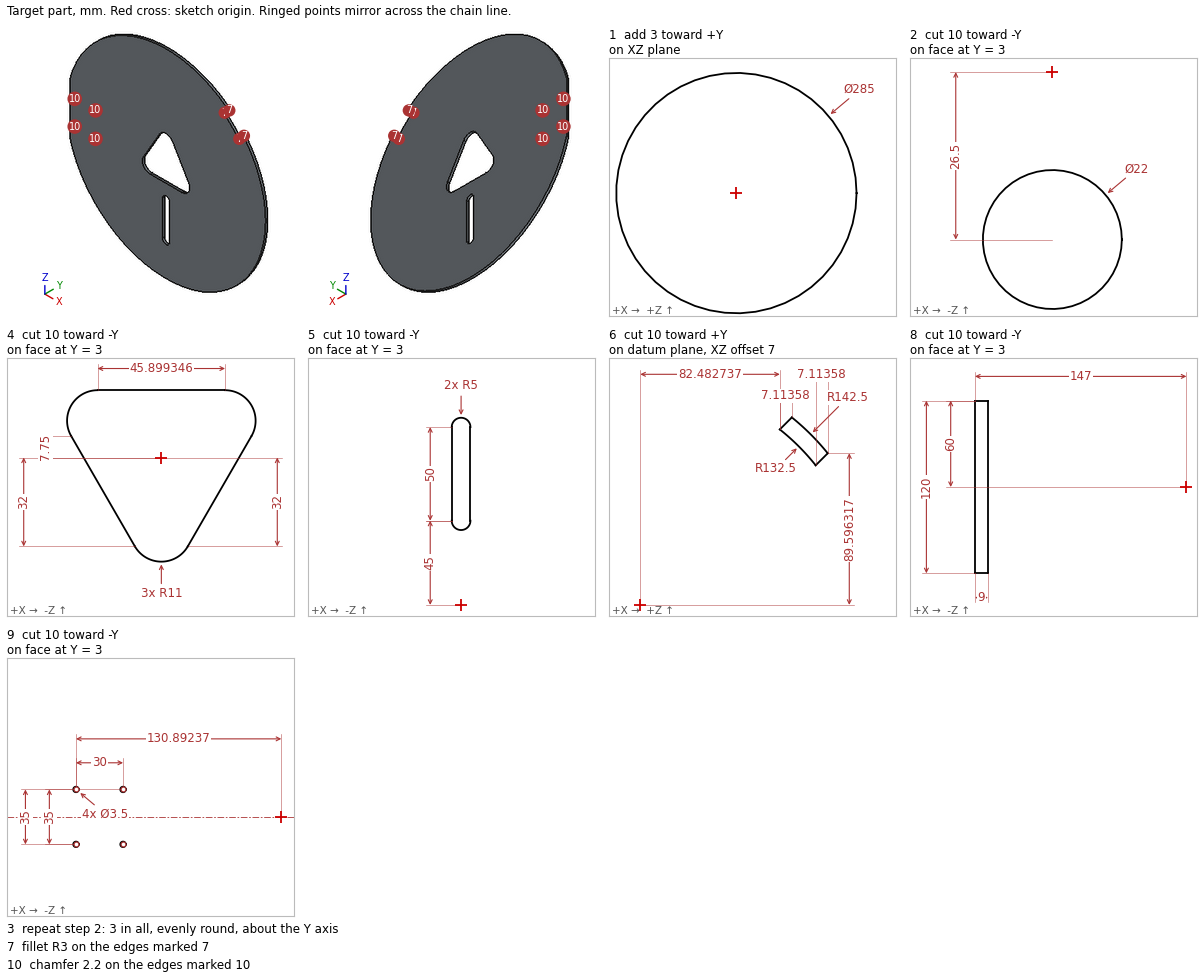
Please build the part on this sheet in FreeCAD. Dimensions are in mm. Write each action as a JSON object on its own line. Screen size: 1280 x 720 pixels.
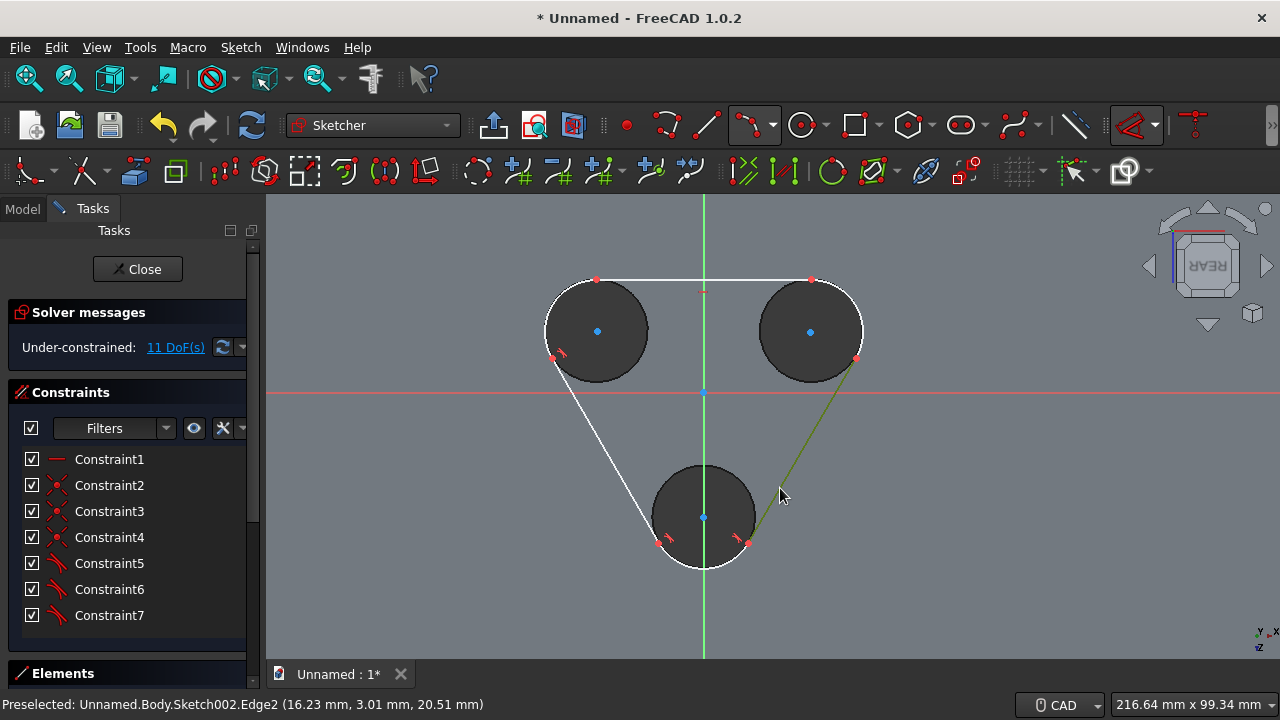
{"action": "left_click", "coordinate": [863, 327]}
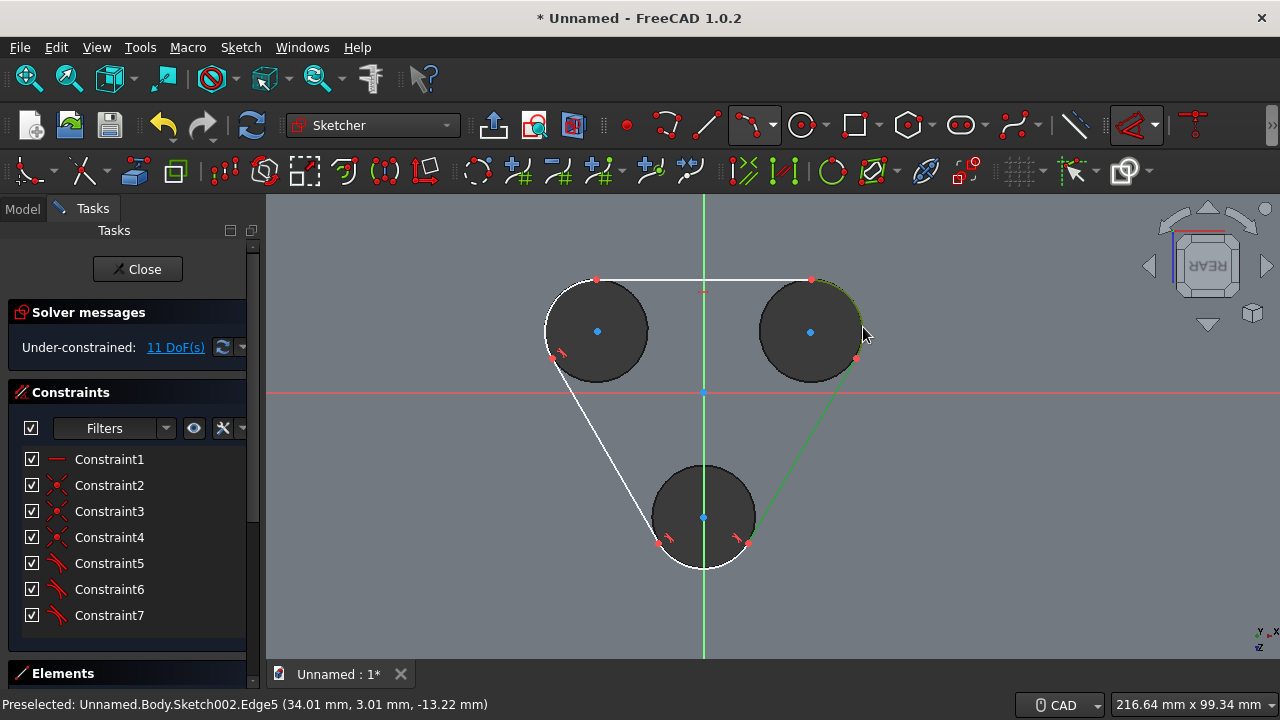
{"action": "key", "text": "t"}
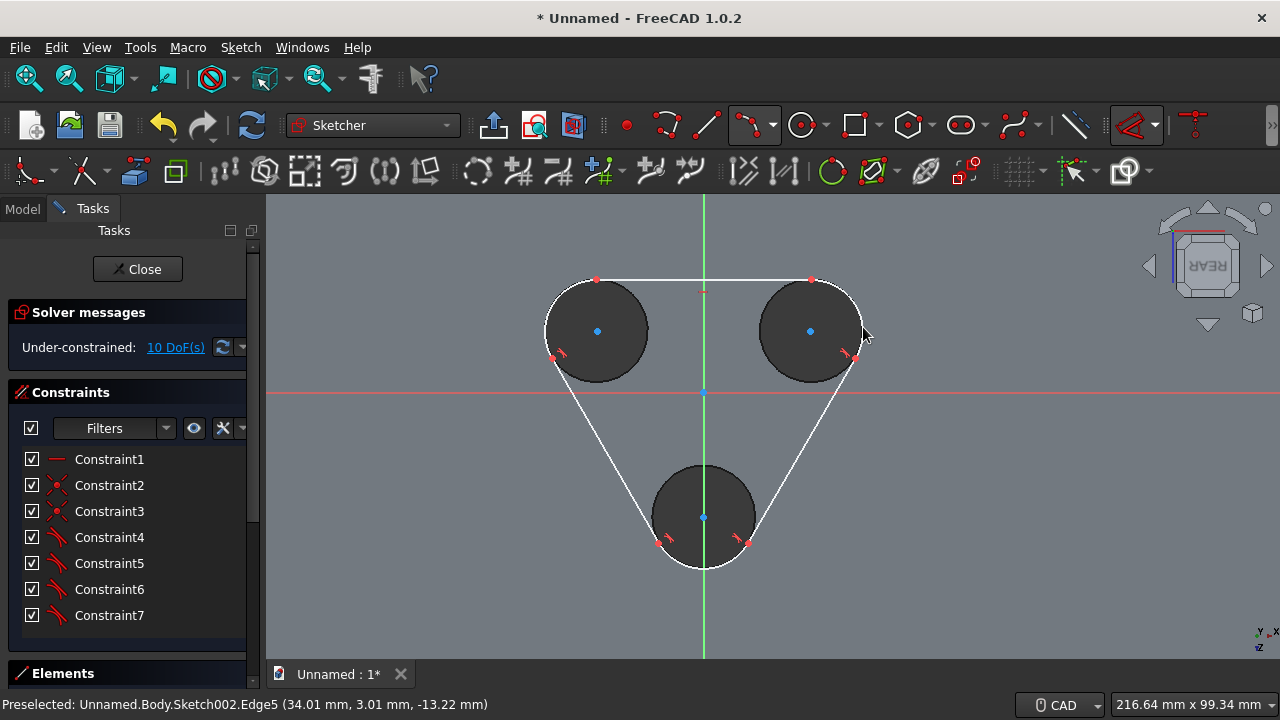
{"action": "left_click", "coordinate": [746, 280]}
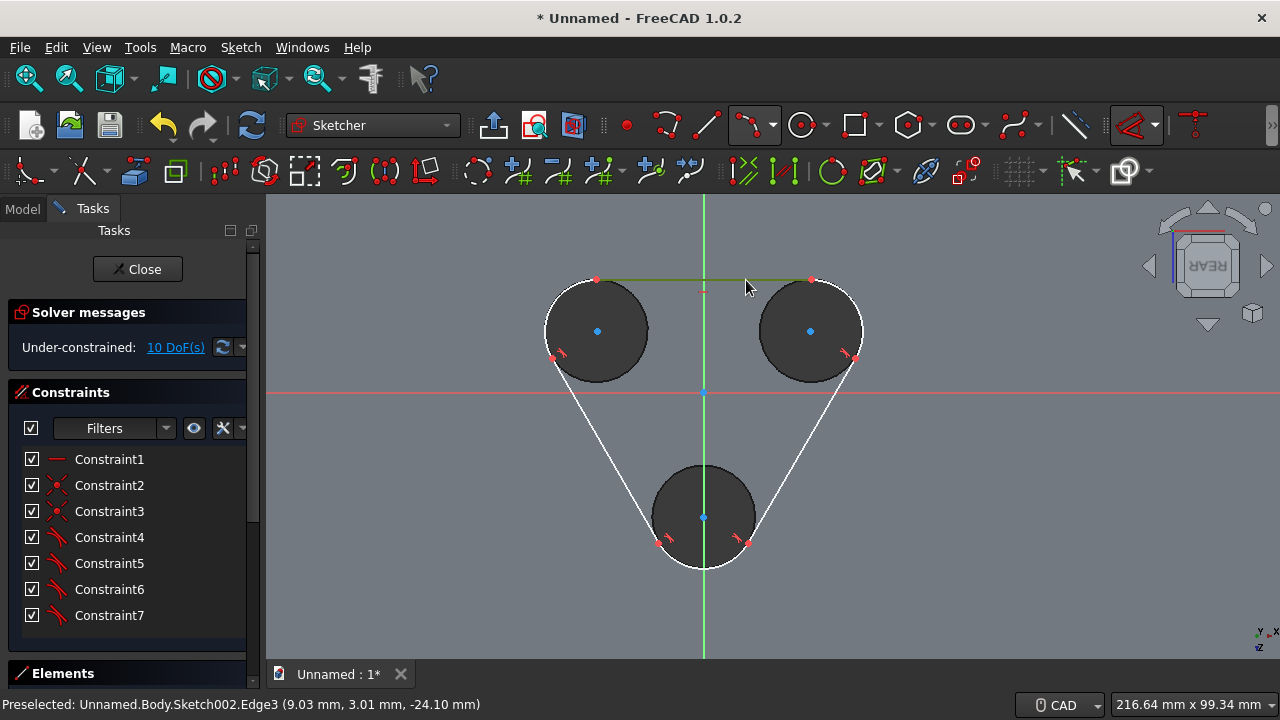
{"action": "left_click", "coordinate": [863, 327]}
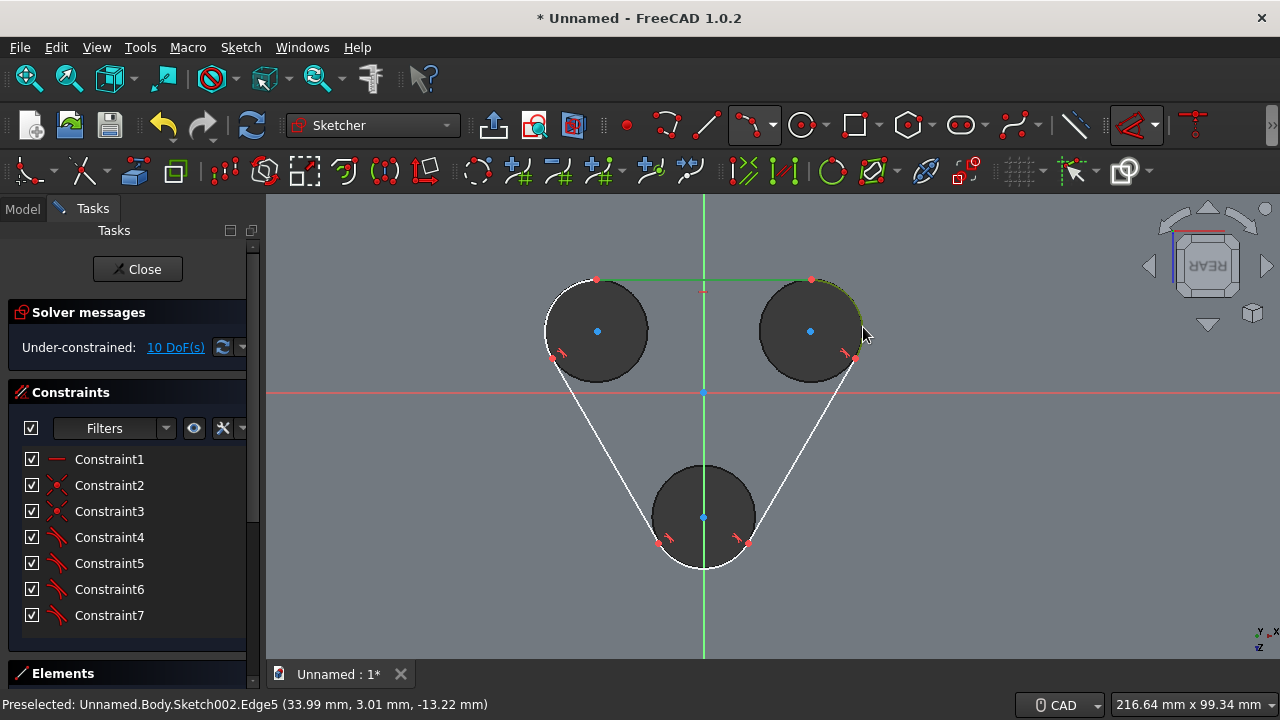
{"action": "key", "text": "t"}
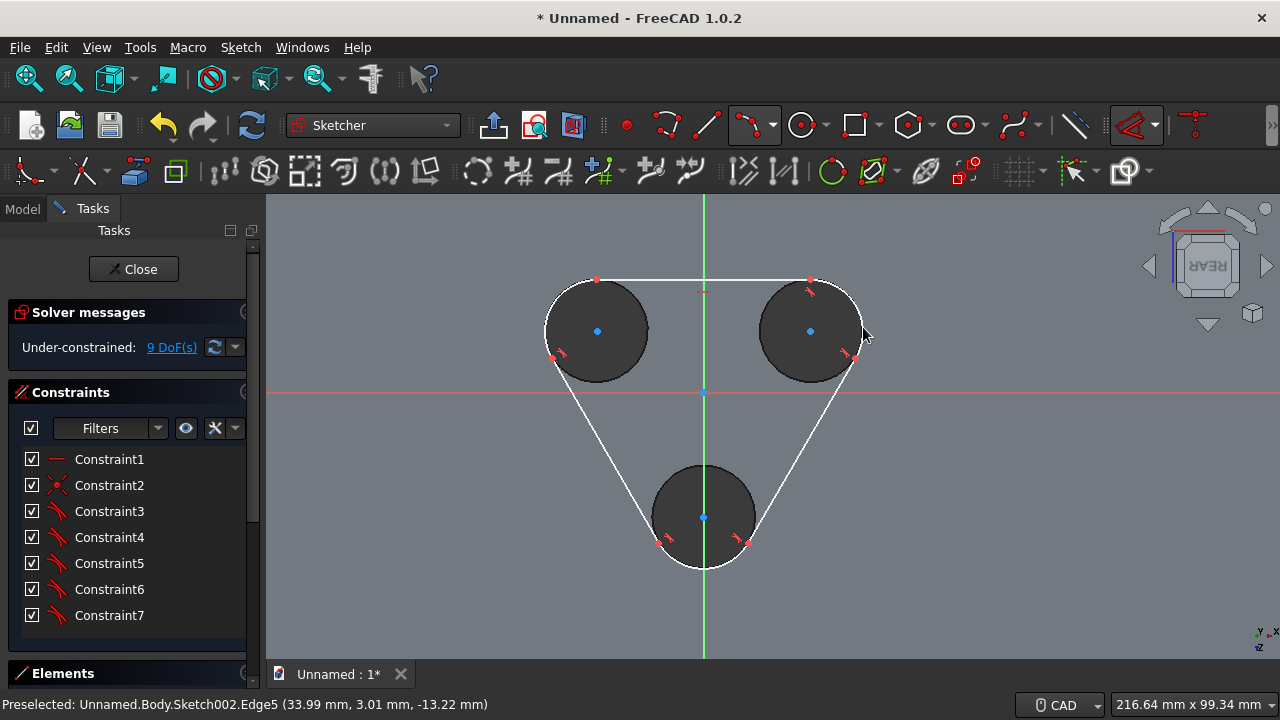
{"action": "left_click", "coordinate": [746, 280]}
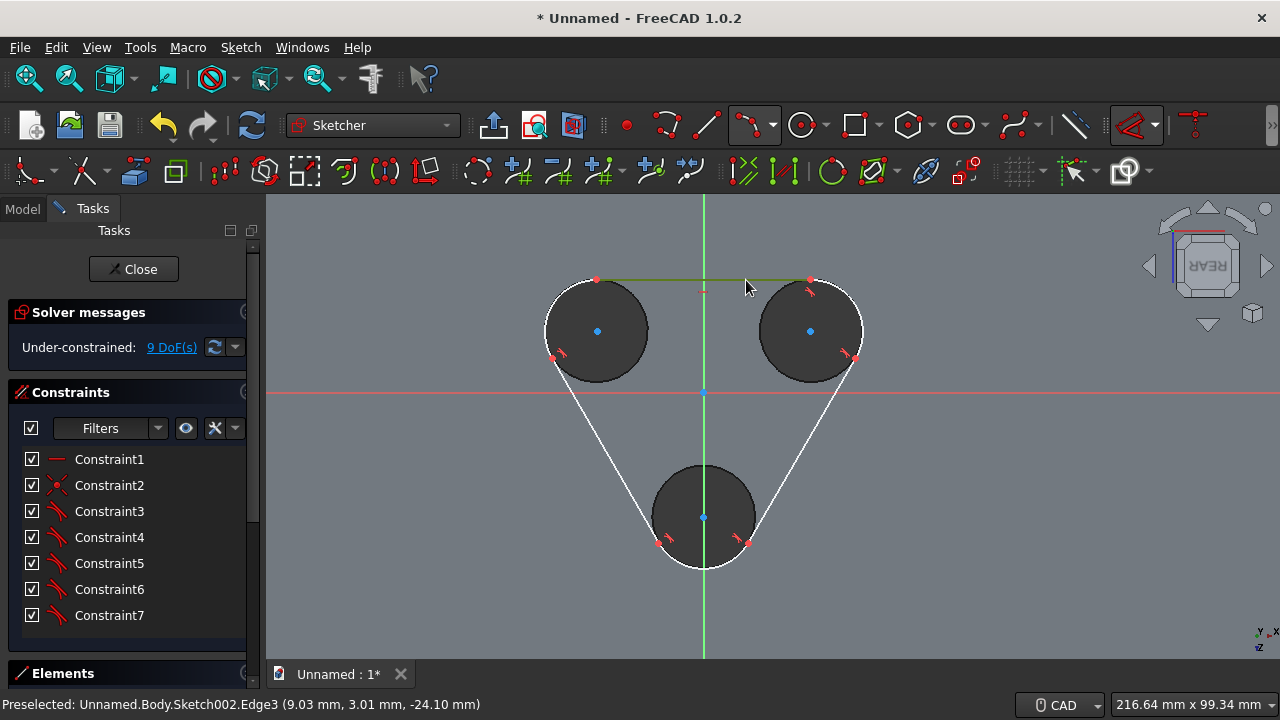
{"action": "left_click", "coordinate": [566, 290]}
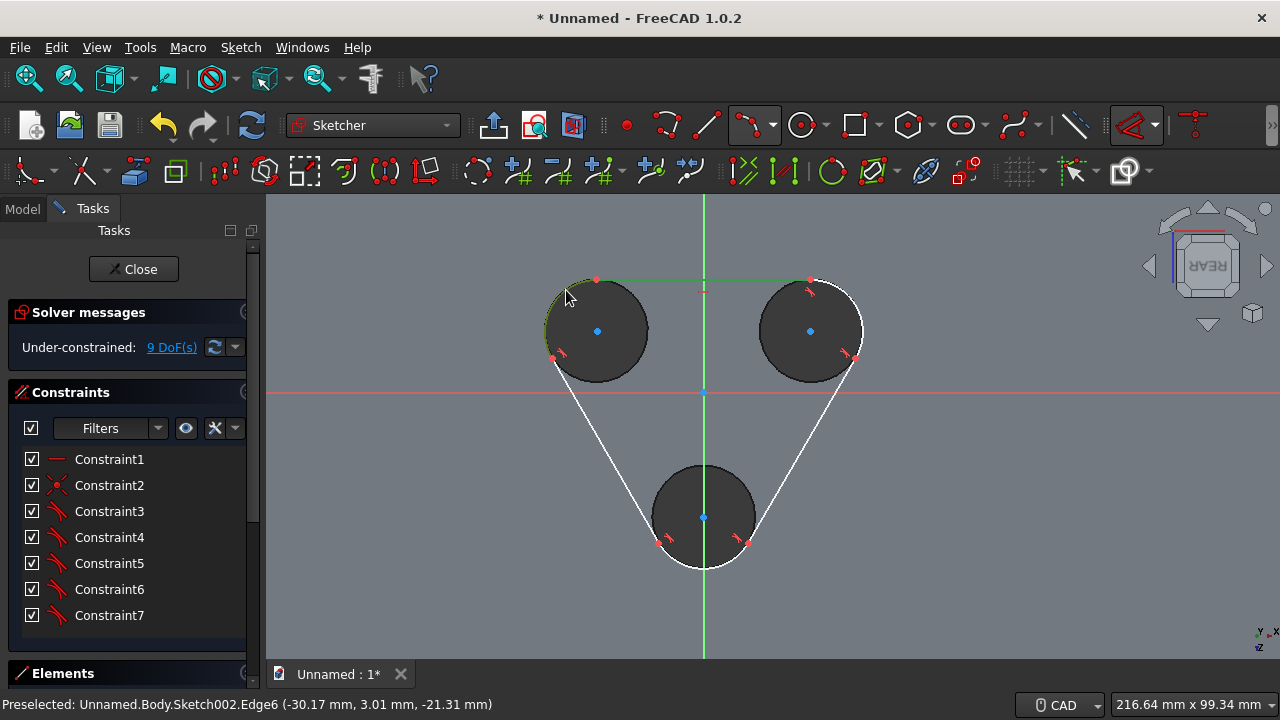
{"action": "key", "text": "t"}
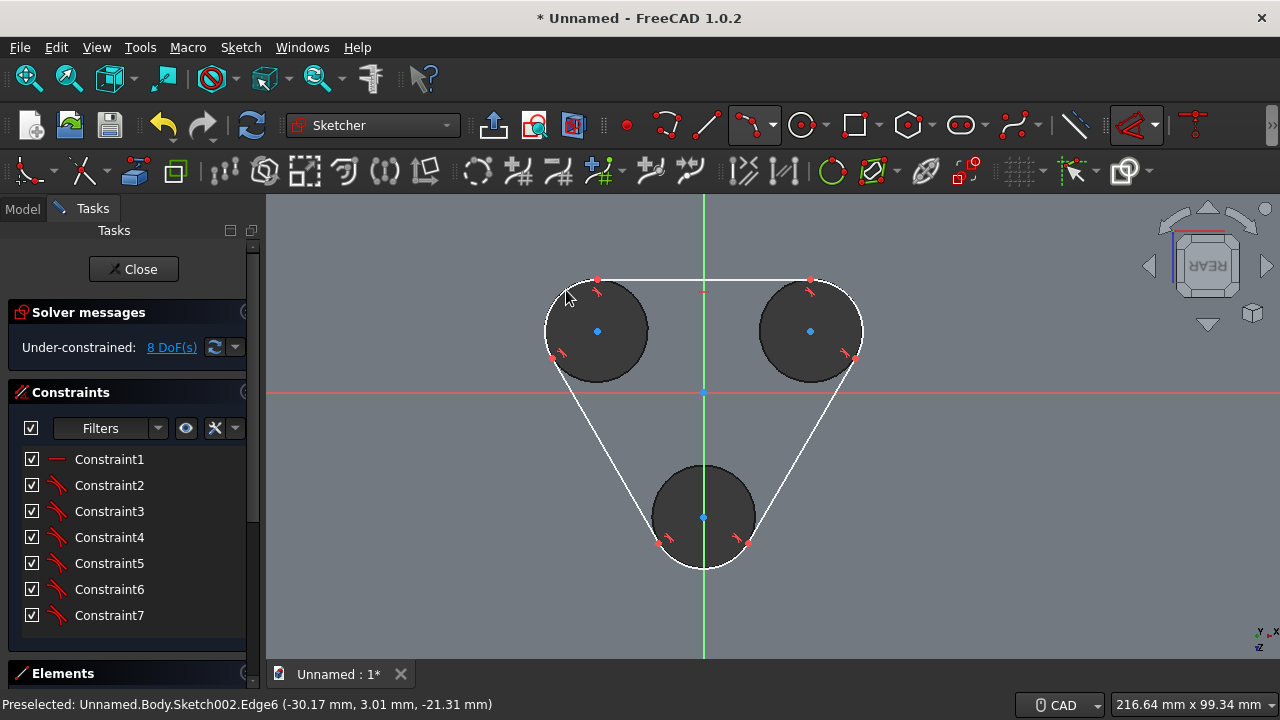
{"action": "left_click", "coordinate": [683, 564]}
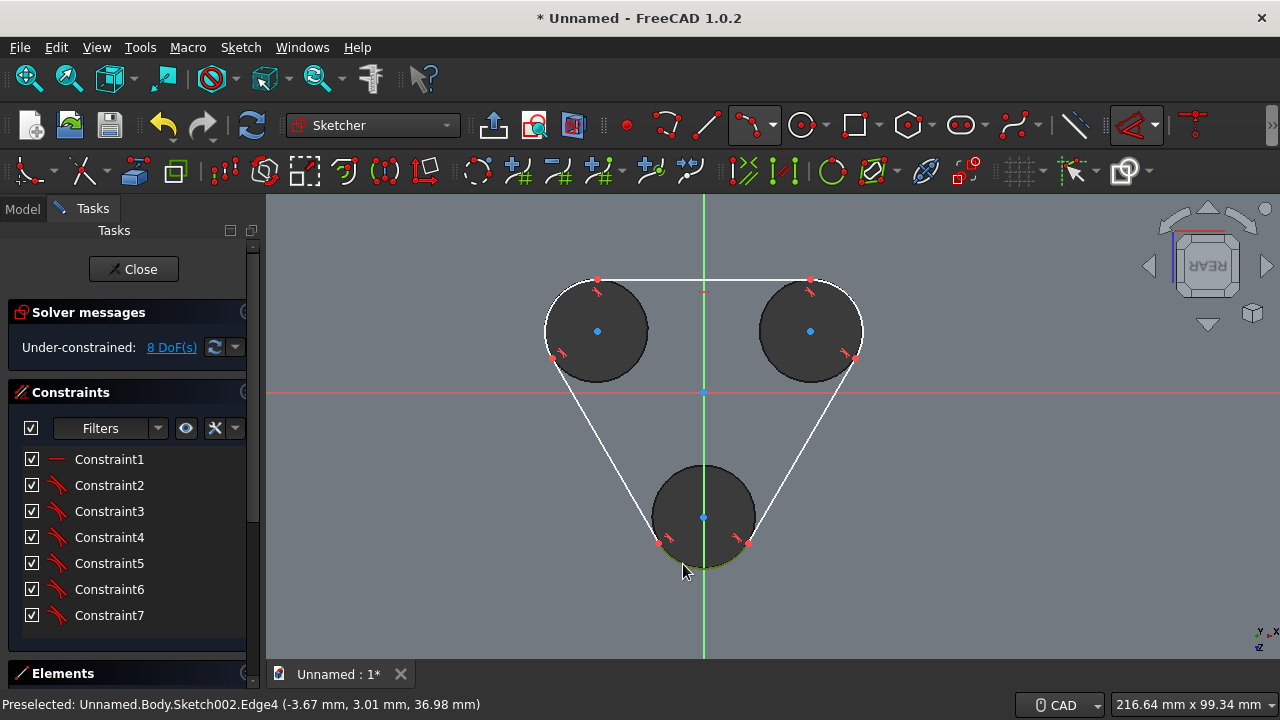
{"action": "left_click", "coordinate": [863, 327]}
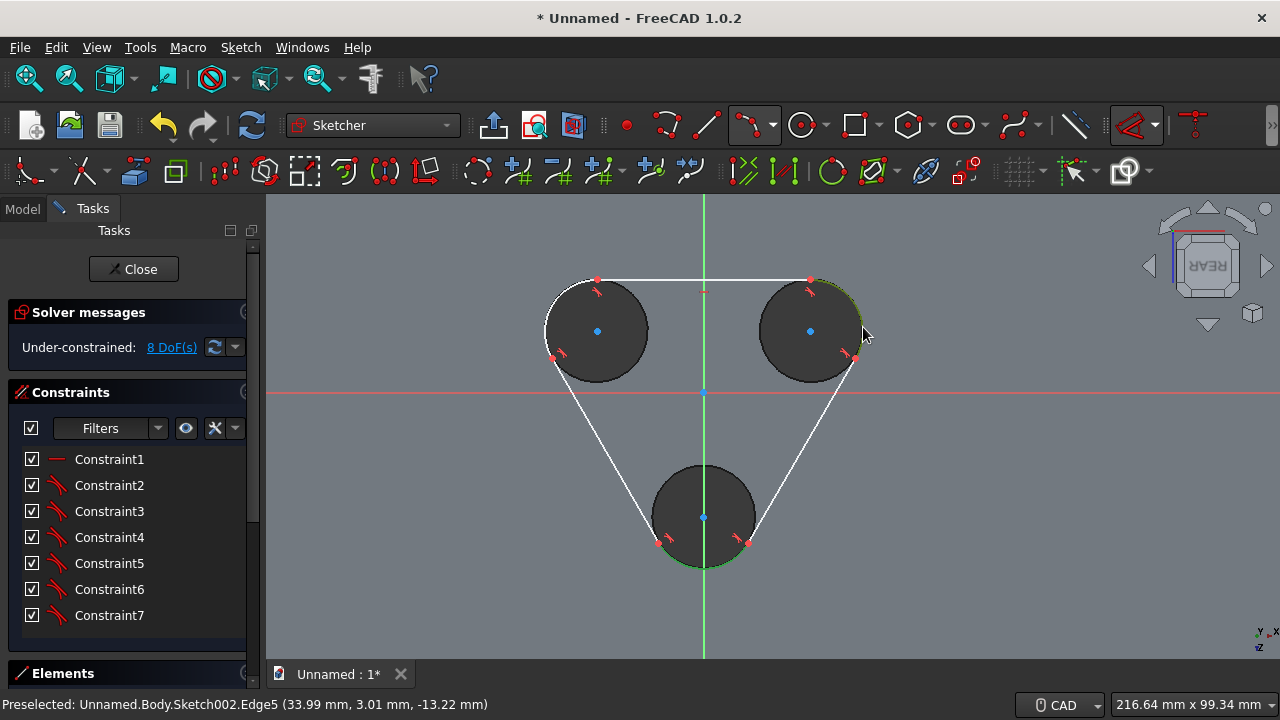
{"action": "left_click", "coordinate": [566, 290]}